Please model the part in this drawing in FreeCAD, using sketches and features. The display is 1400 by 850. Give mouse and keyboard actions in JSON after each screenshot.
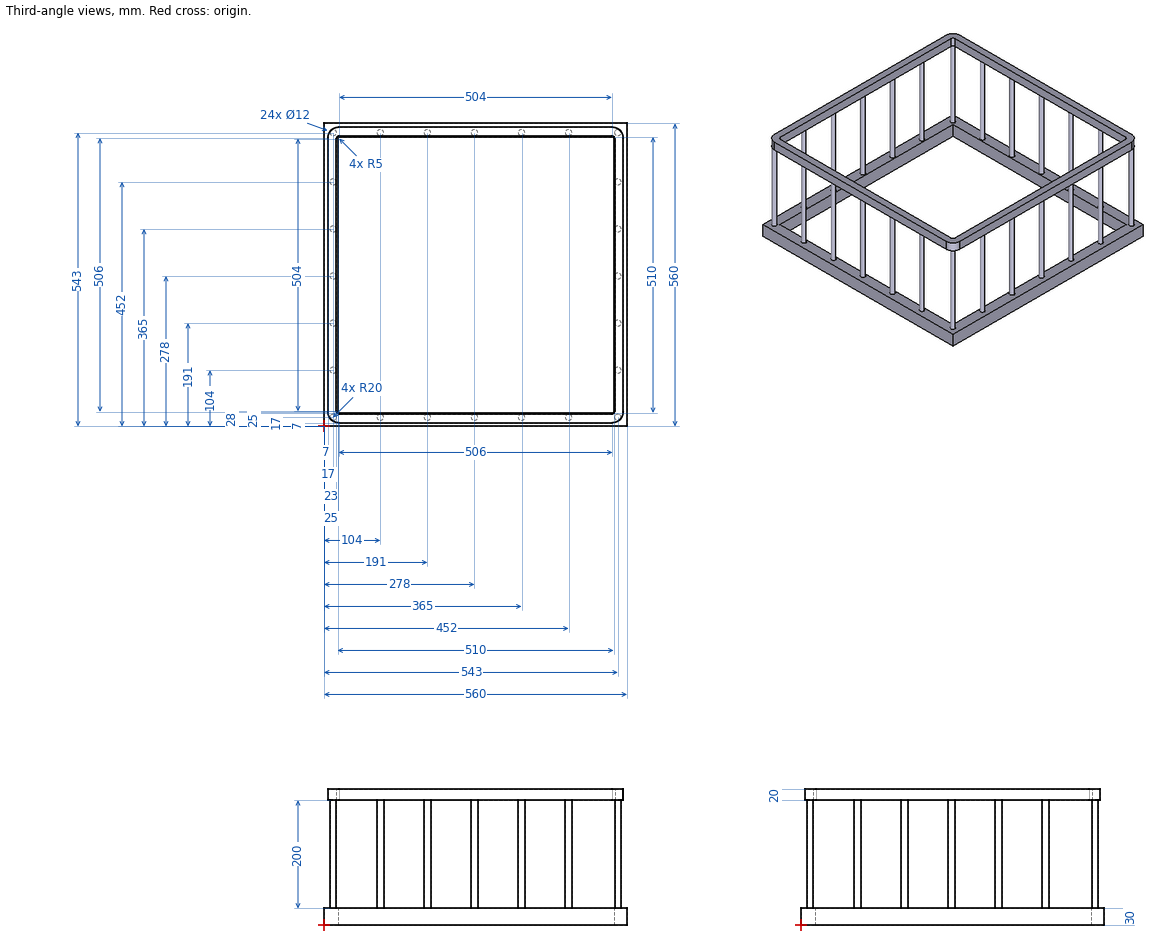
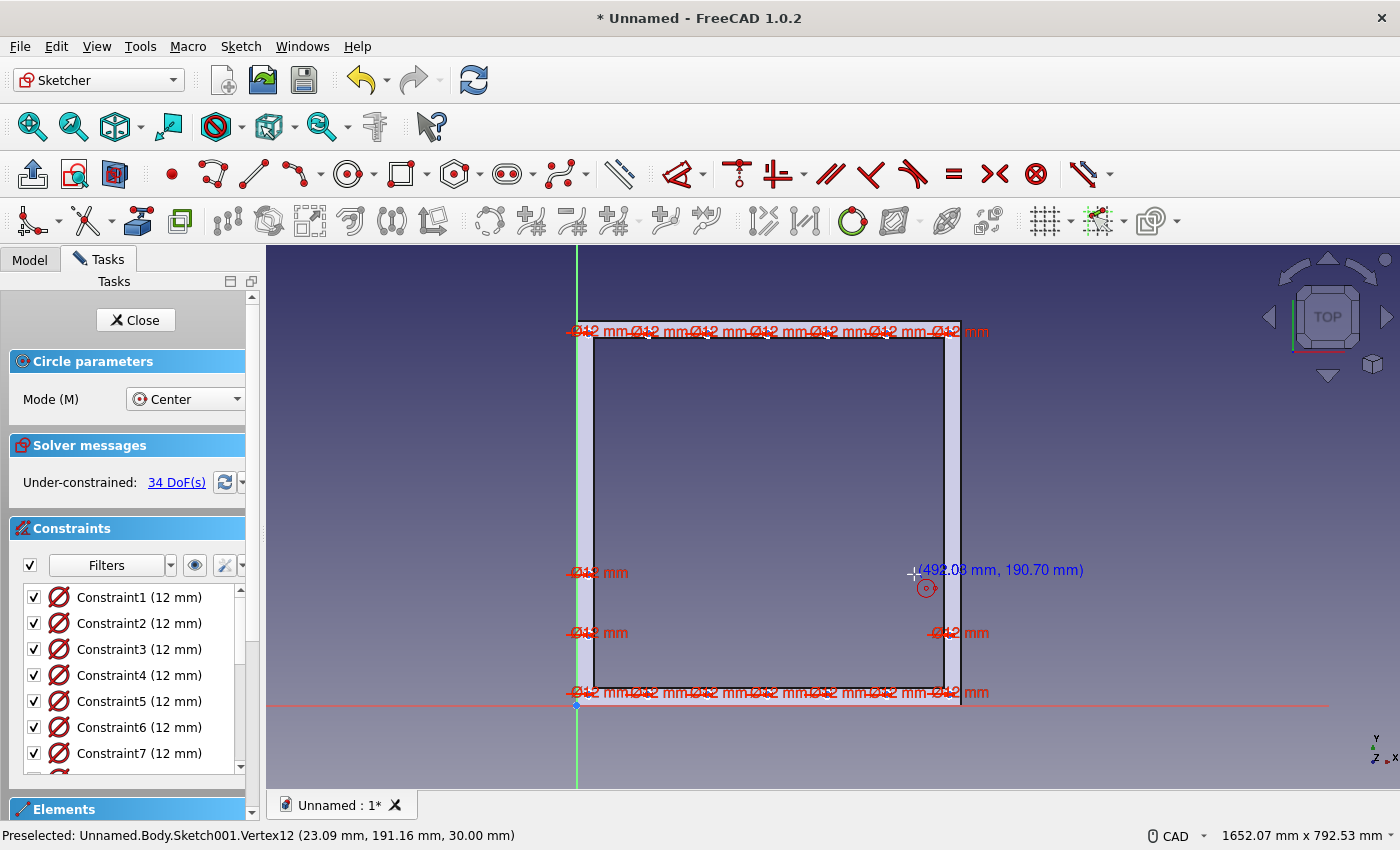
{"action": "left_click", "coordinate": [949, 574]}
{"action": "mouse_move", "coordinate": [952, 572]}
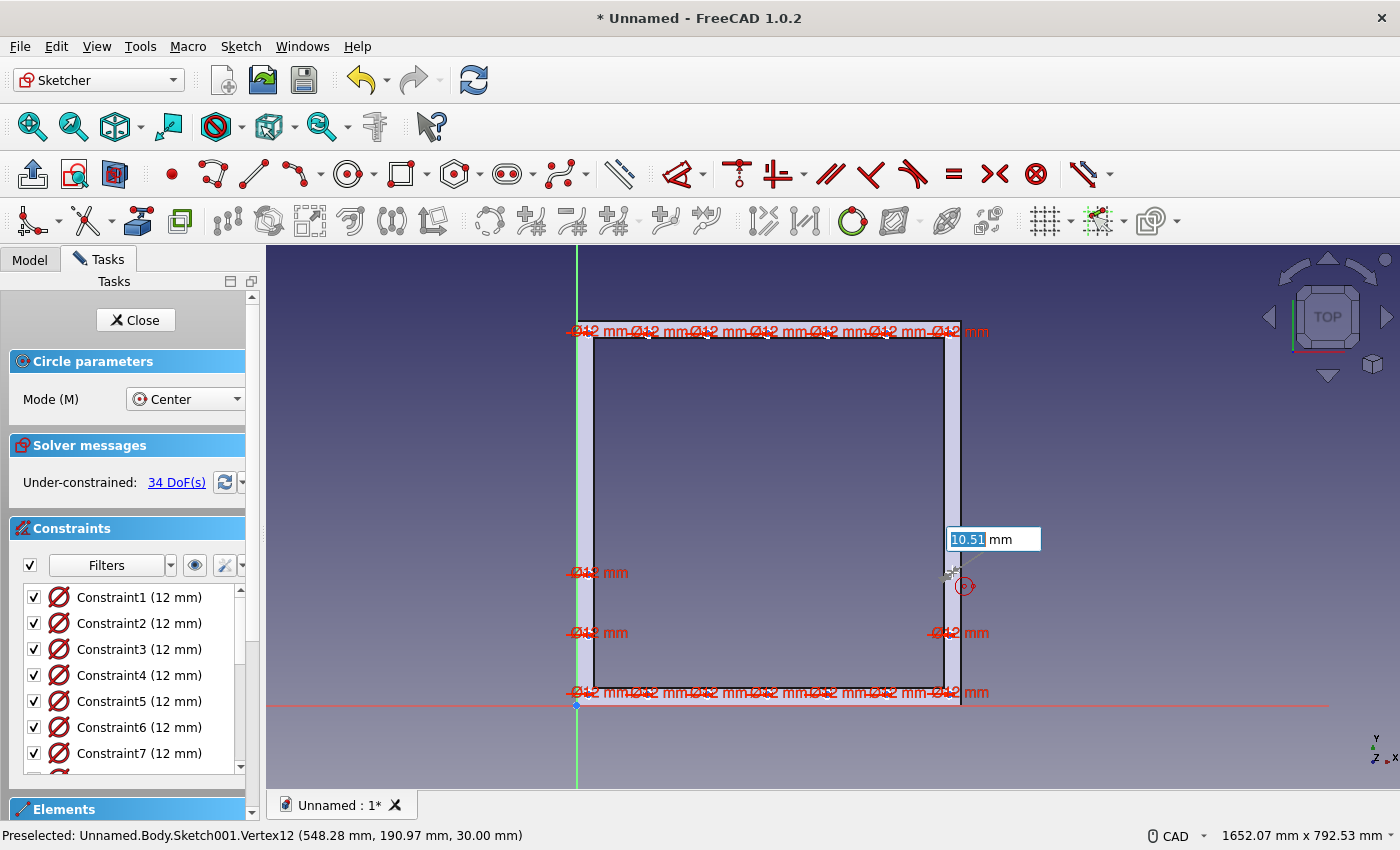
{"action": "type", "text": "12"}
{"action": "key", "text": "Return"}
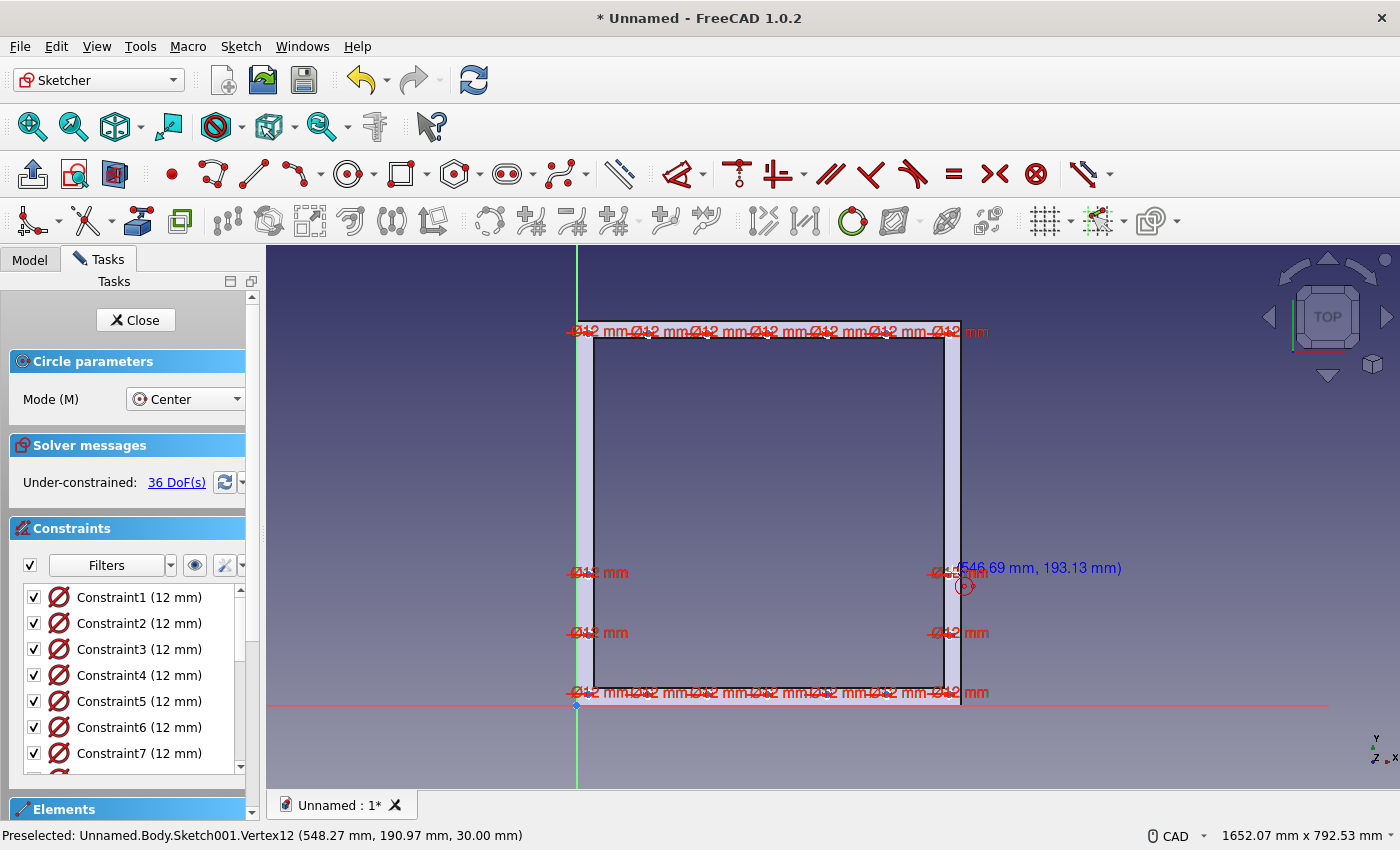
{"action": "scroll", "coordinate": [588, 515], "scroll_direction": "up", "scroll_amount": 9}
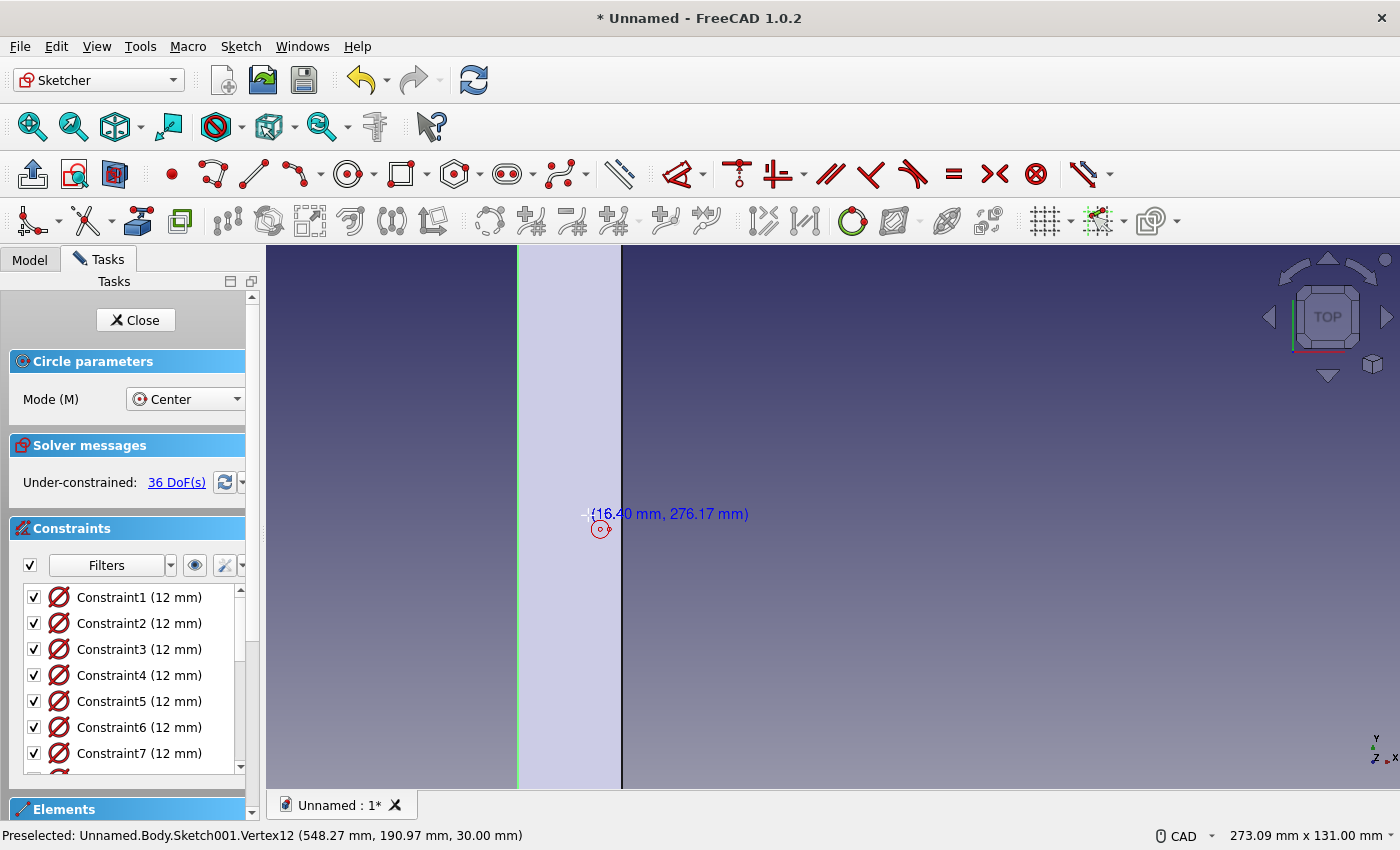
{"action": "scroll", "coordinate": [587, 515], "scroll_direction": "down", "scroll_amount": 9}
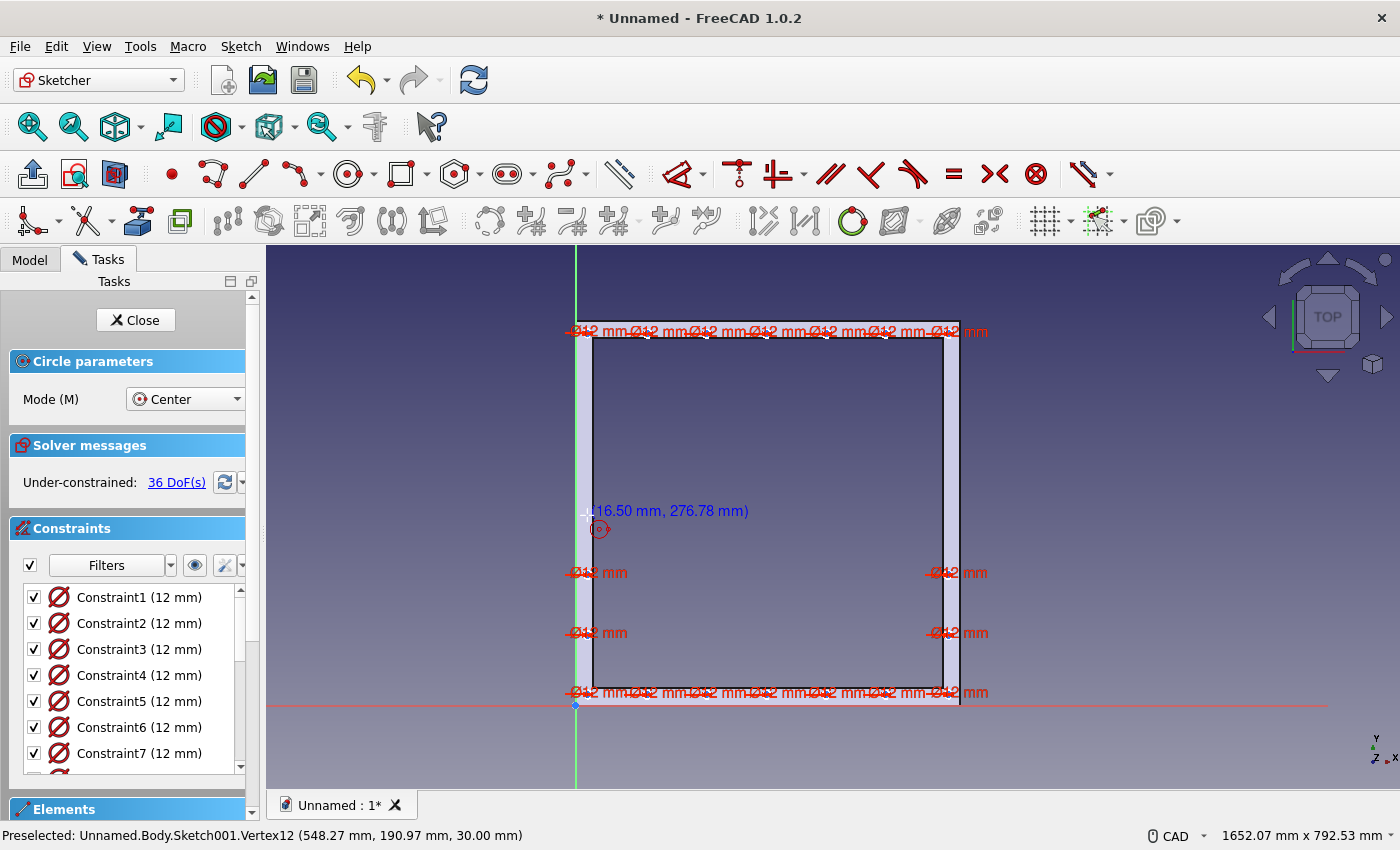
{"action": "scroll", "coordinate": [588, 515], "scroll_direction": "up", "scroll_amount": 2}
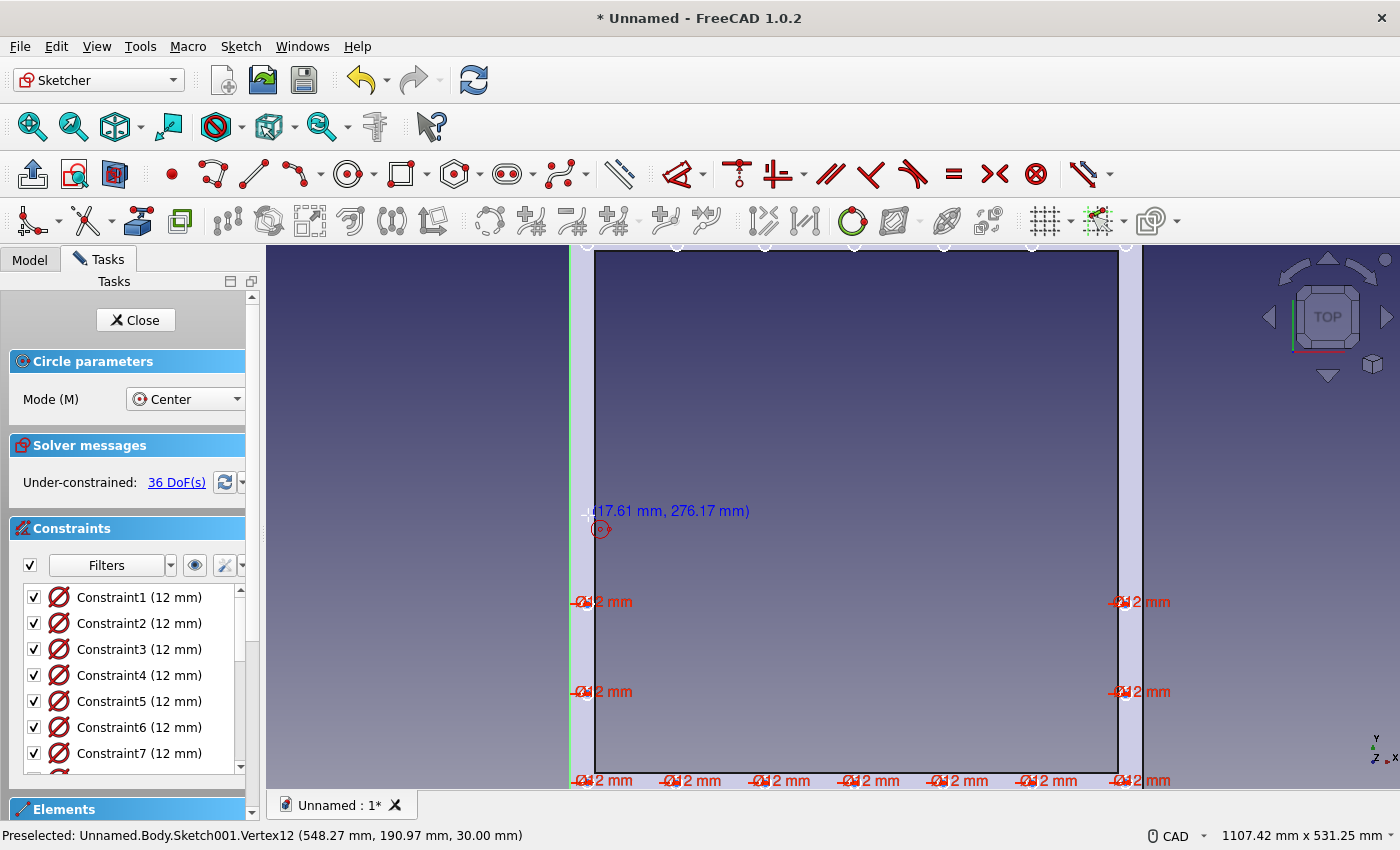
{"action": "left_click", "coordinate": [587, 514]}
{"action": "mouse_move", "coordinate": [592, 510]}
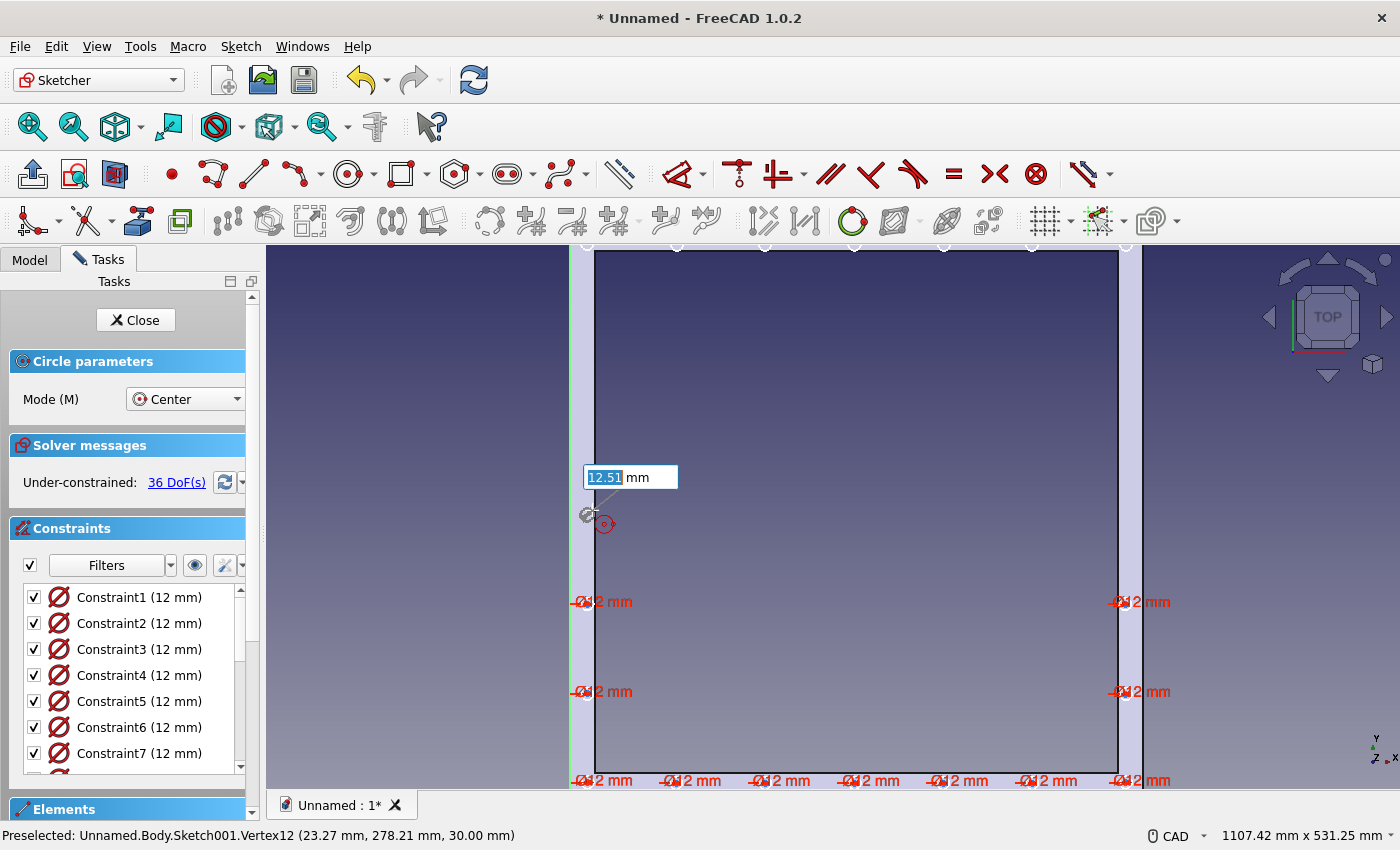
{"action": "type", "text": "12"}
{"action": "key", "text": "Return"}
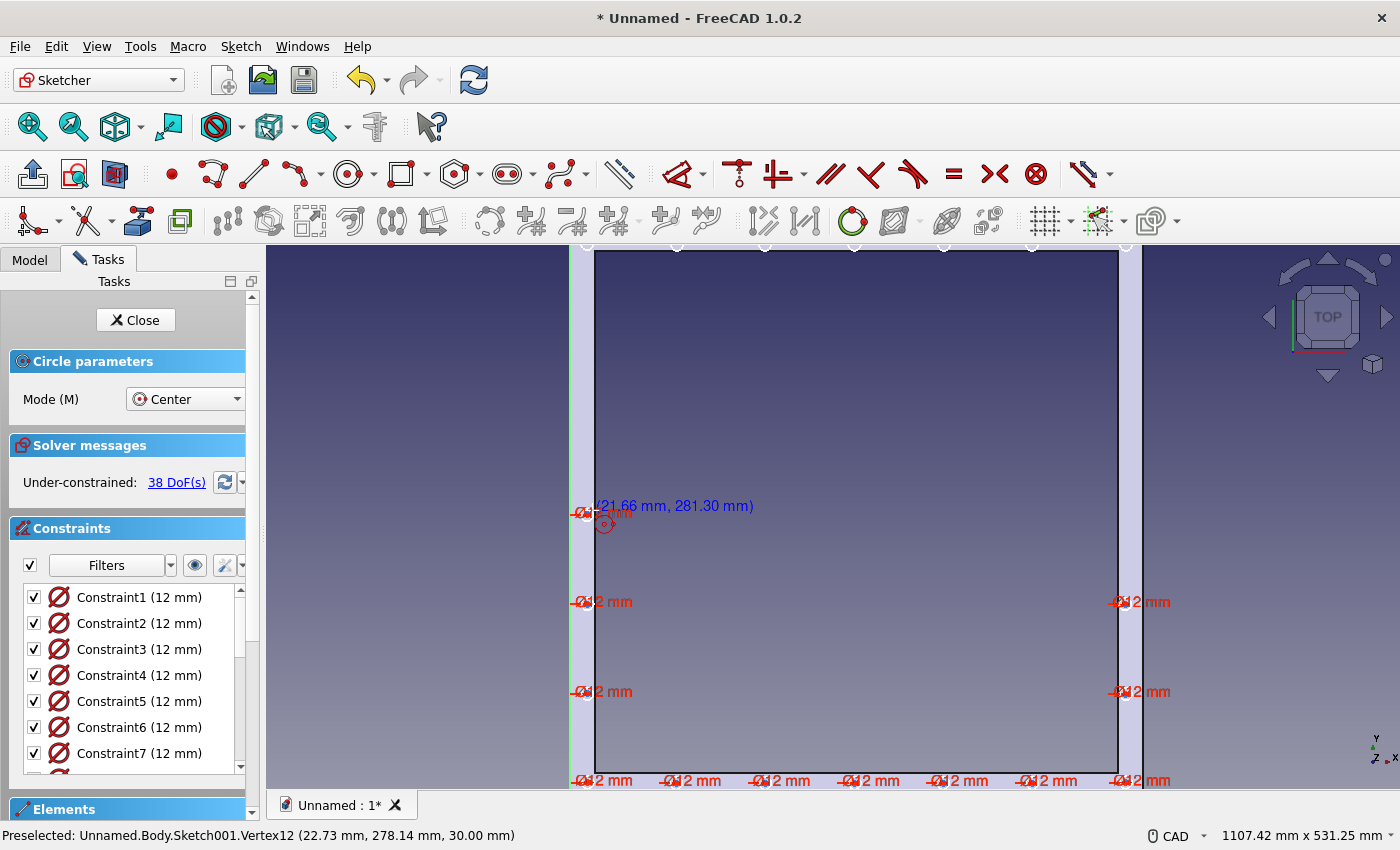
{"action": "scroll", "coordinate": [1126, 514], "scroll_direction": "up", "scroll_amount": 7}